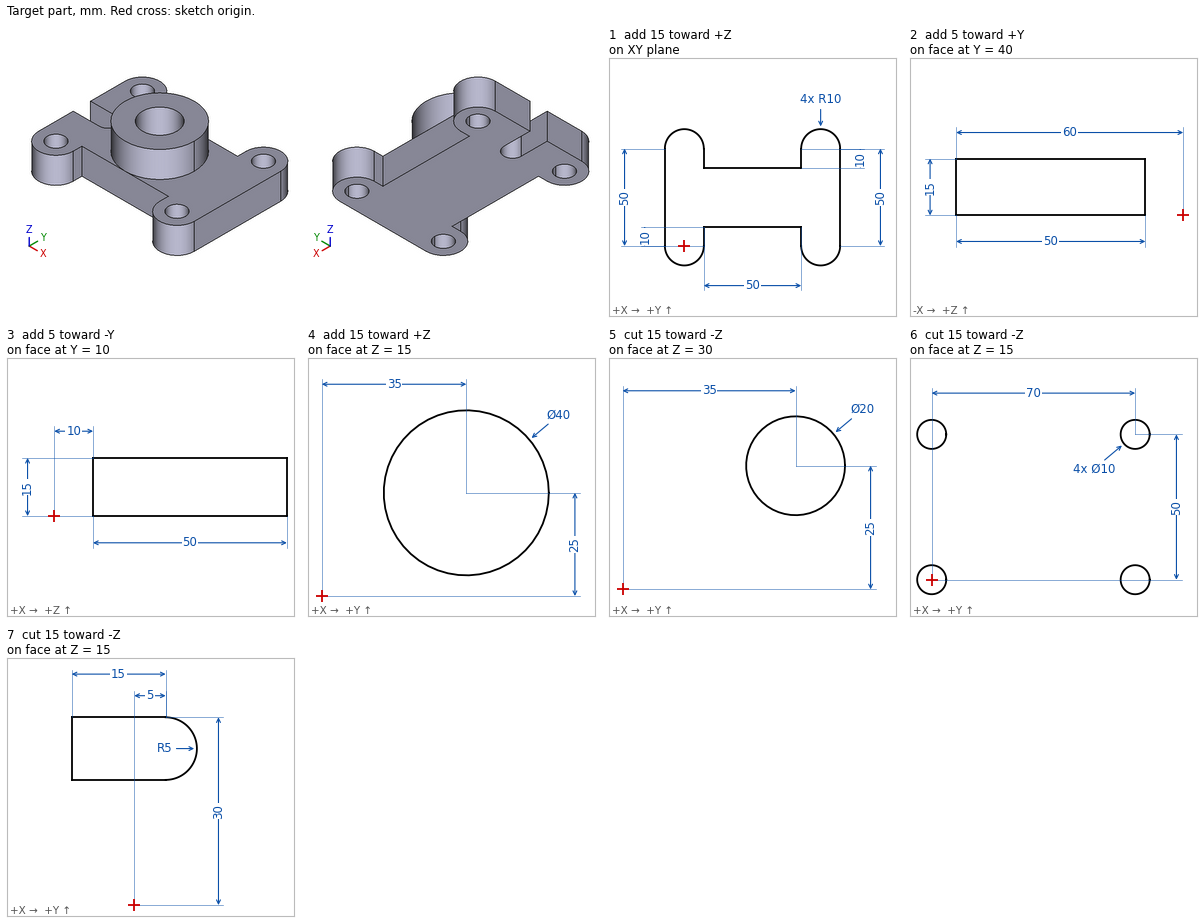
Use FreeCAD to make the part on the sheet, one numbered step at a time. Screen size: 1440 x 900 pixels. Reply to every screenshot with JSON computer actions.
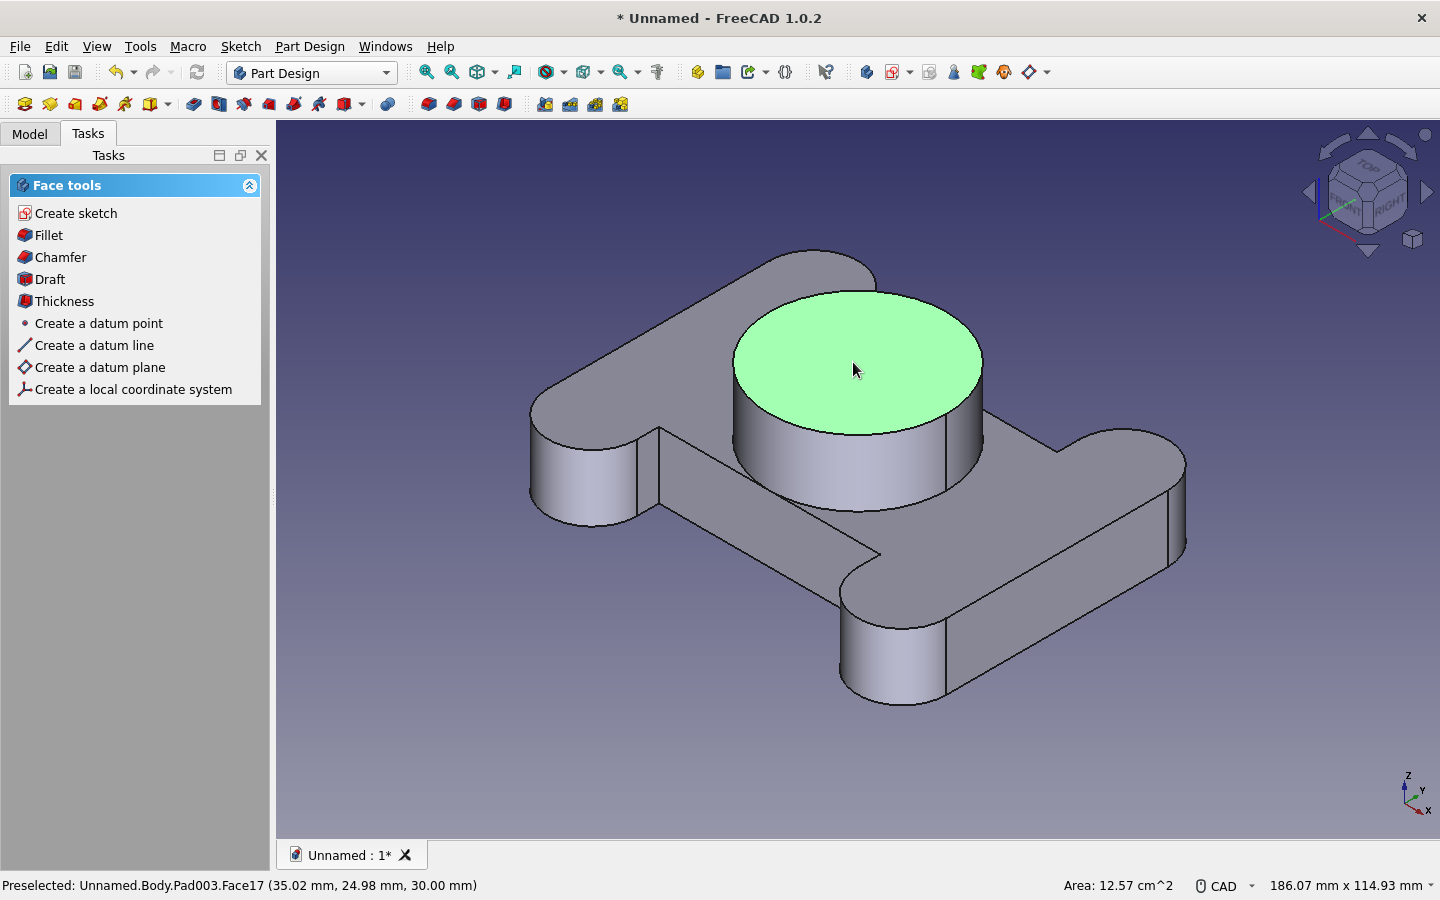
{"action": "left_click", "coordinate": [892, 72]}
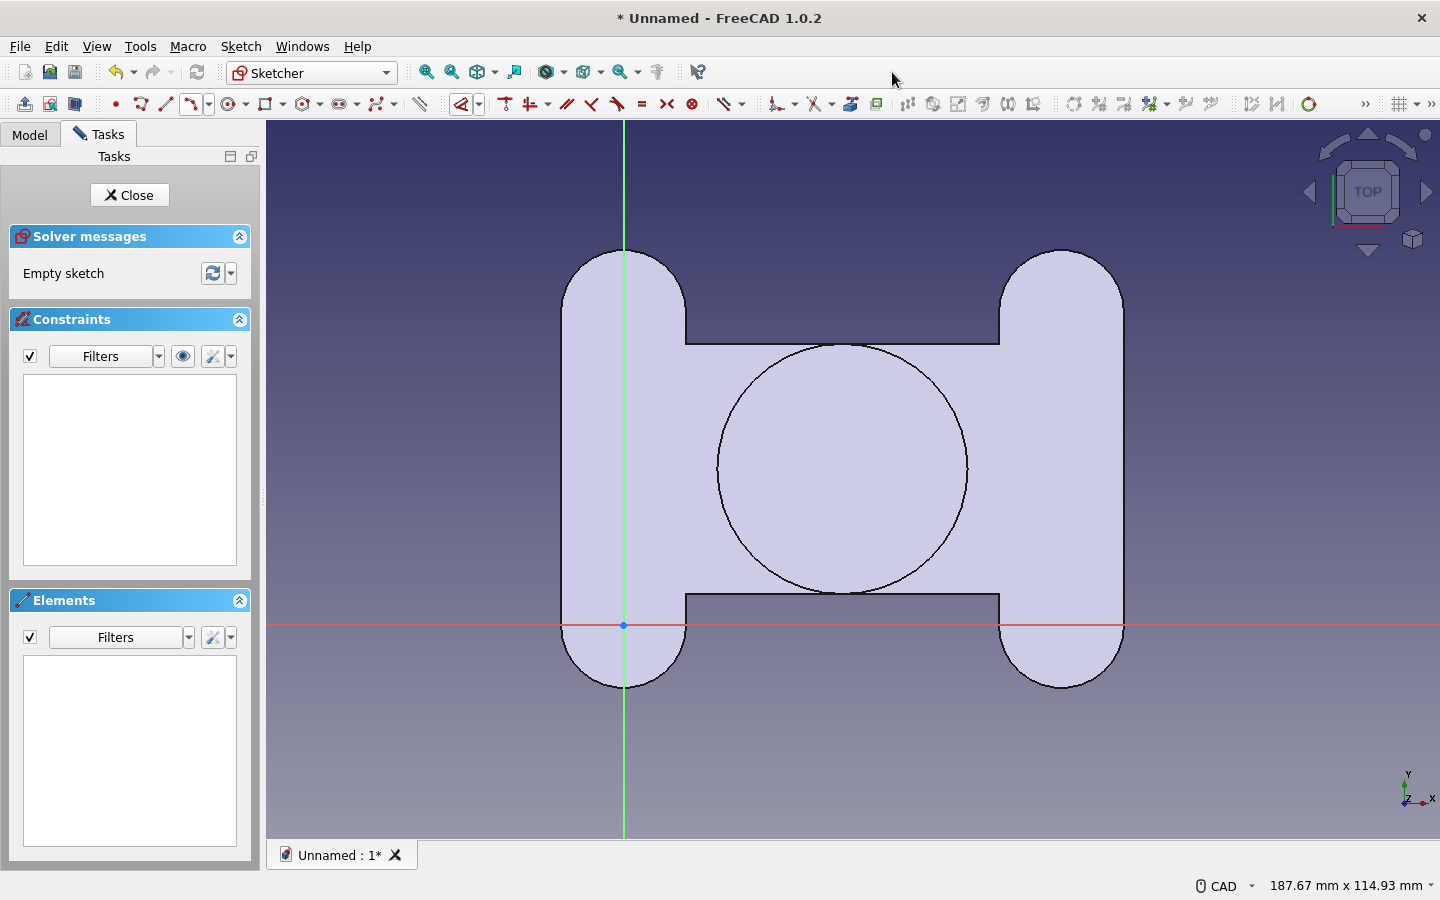
{"action": "scroll", "coordinate": [748, 546], "scroll_direction": "up", "scroll_amount": 4}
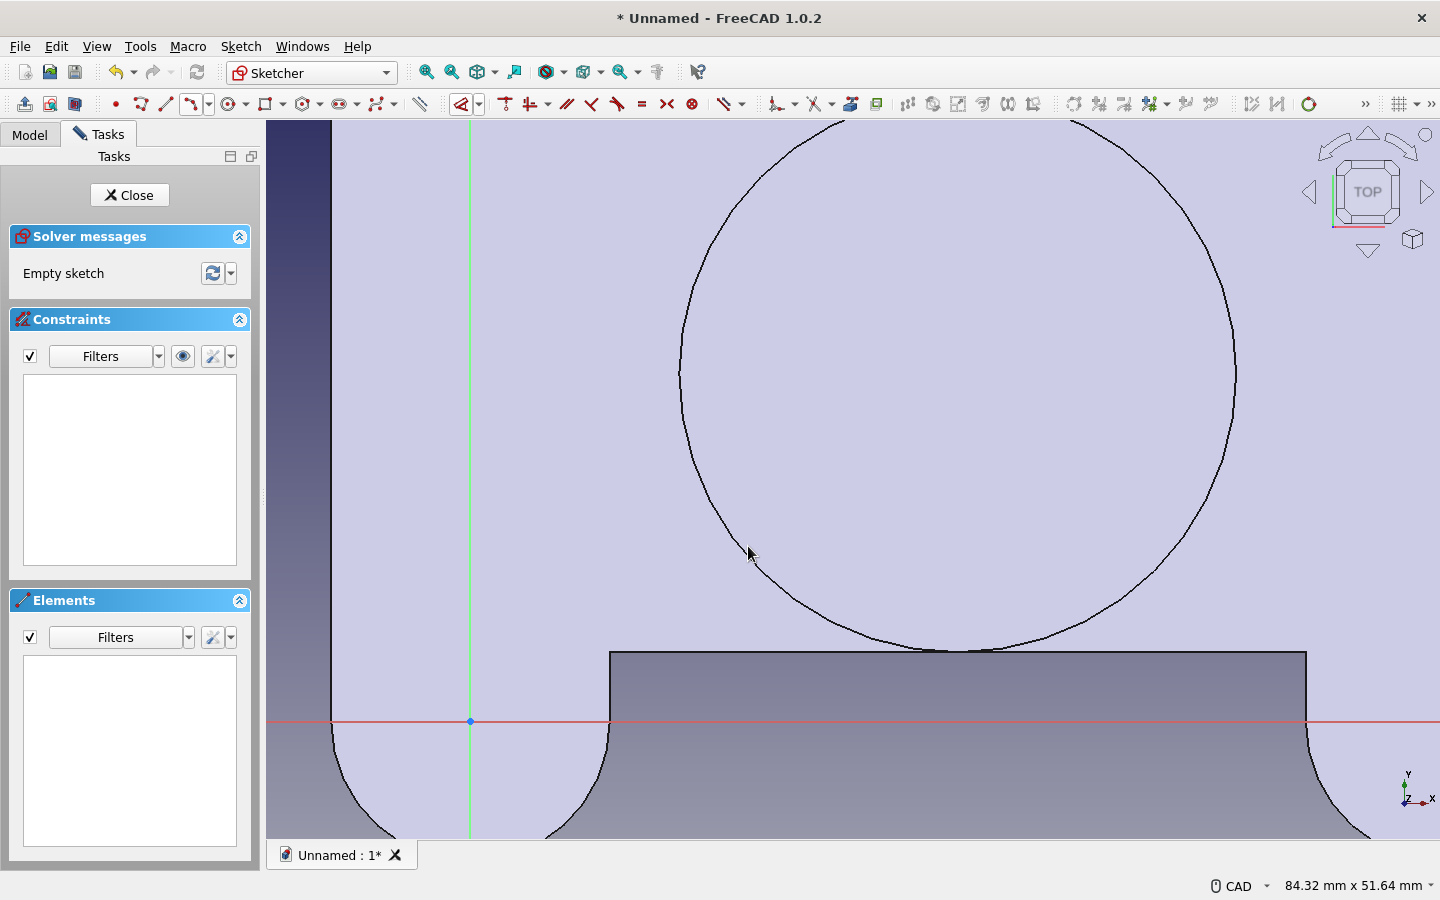
{"action": "key", "text": "g c"}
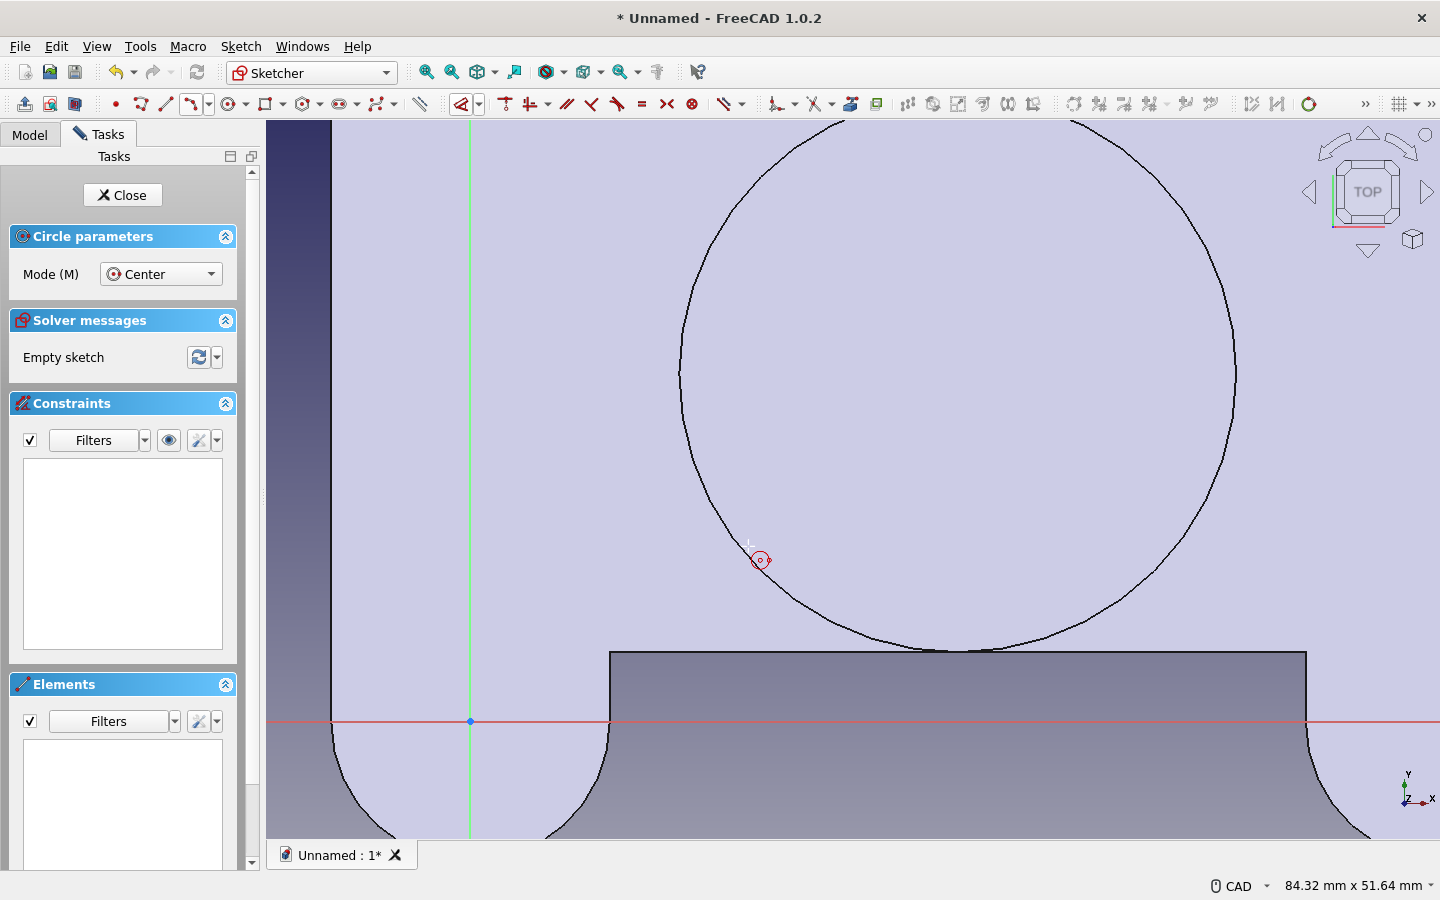
{"action": "left_click", "coordinate": [958, 374]}
{"action": "left_click", "coordinate": [1056, 275]}
{"action": "key", "text": "Escape"}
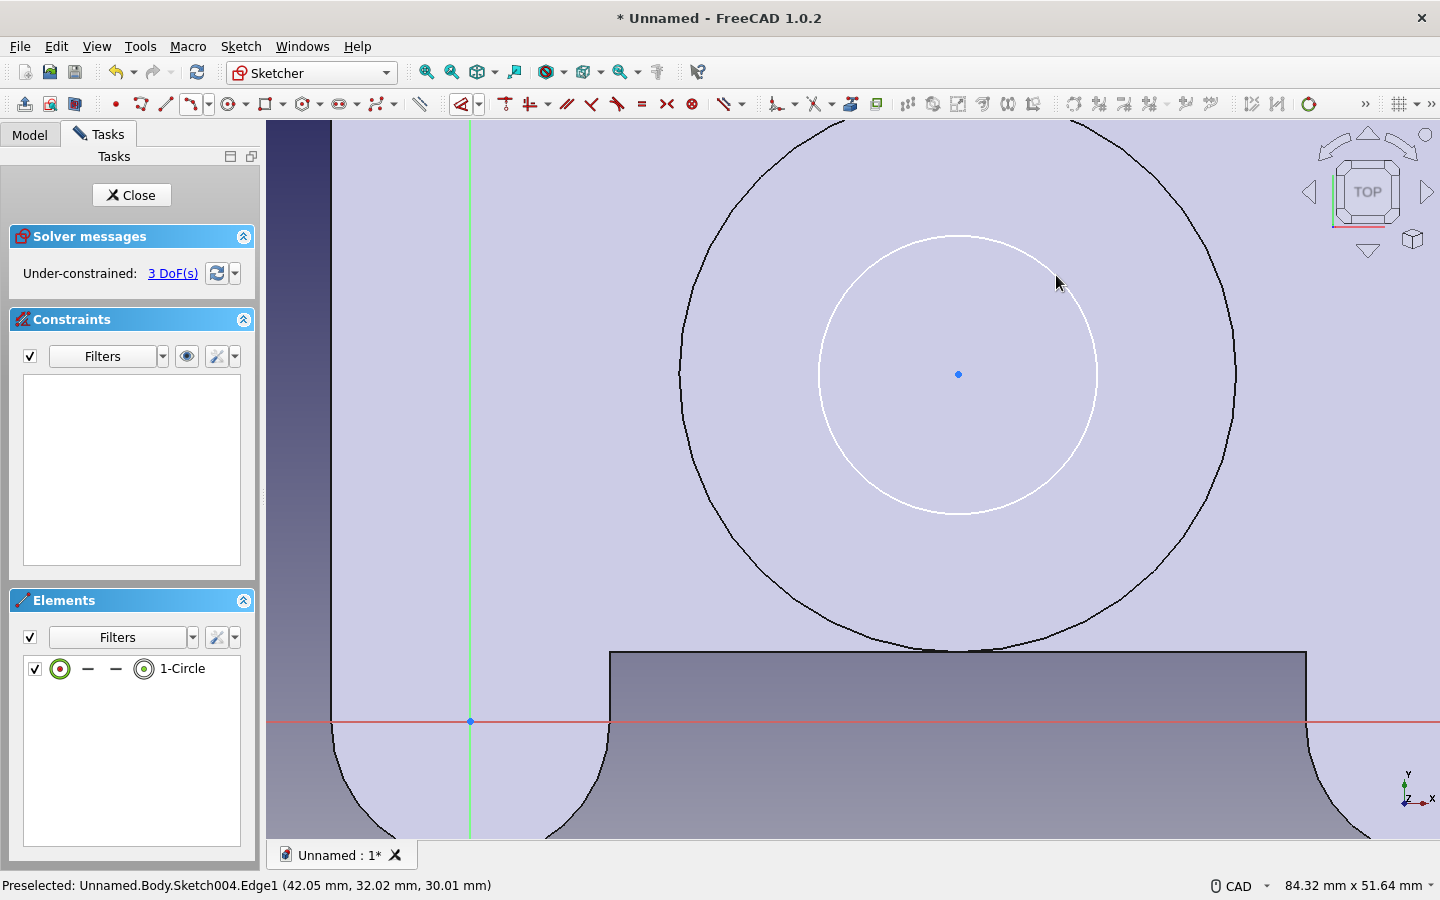
{"action": "left_click", "coordinate": [1056, 276]}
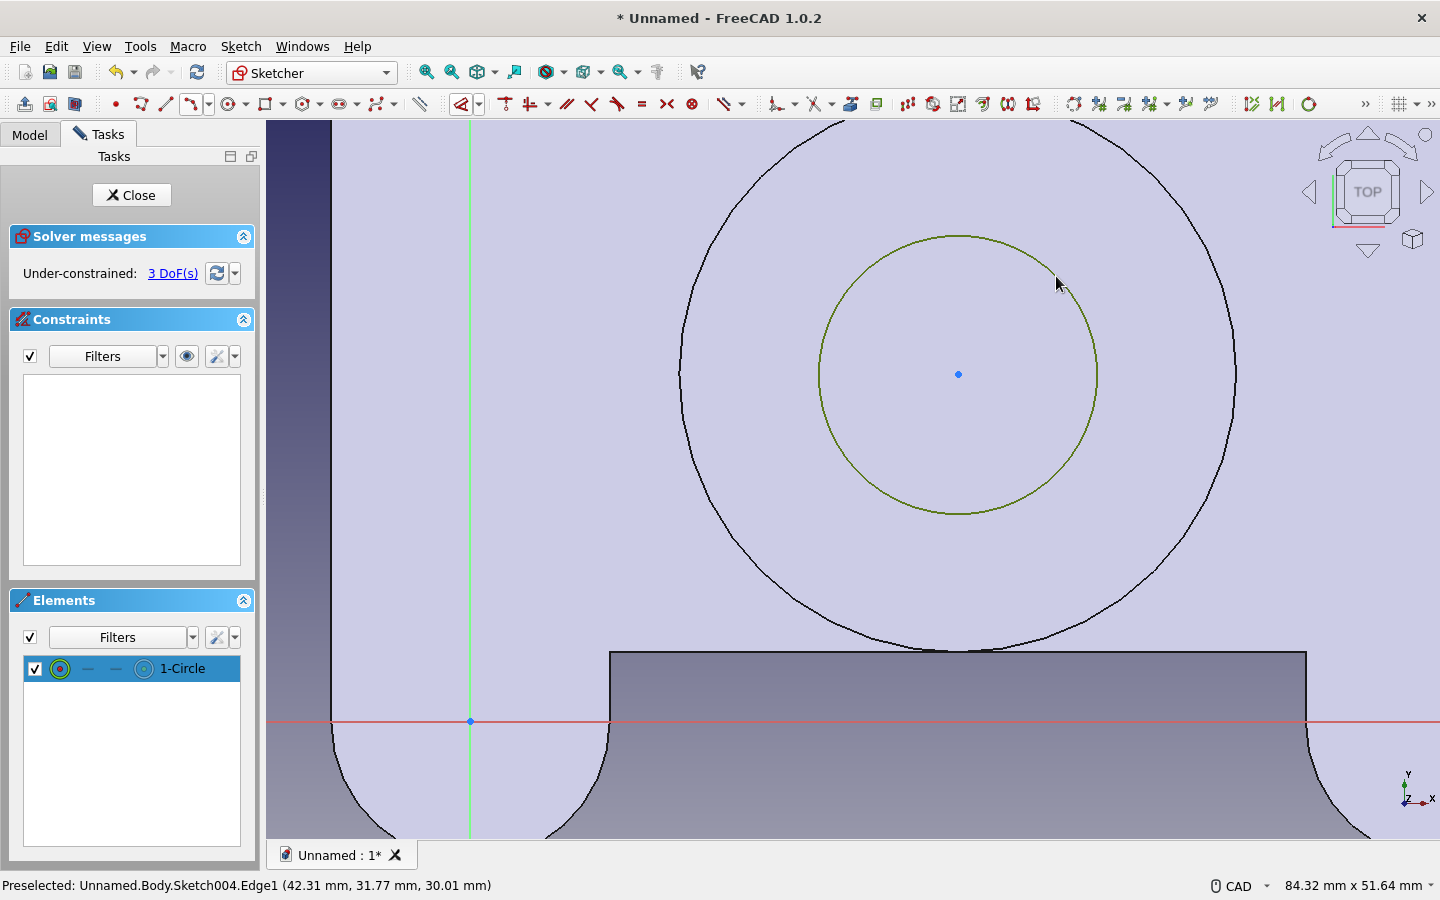
{"action": "key", "text": "k o"}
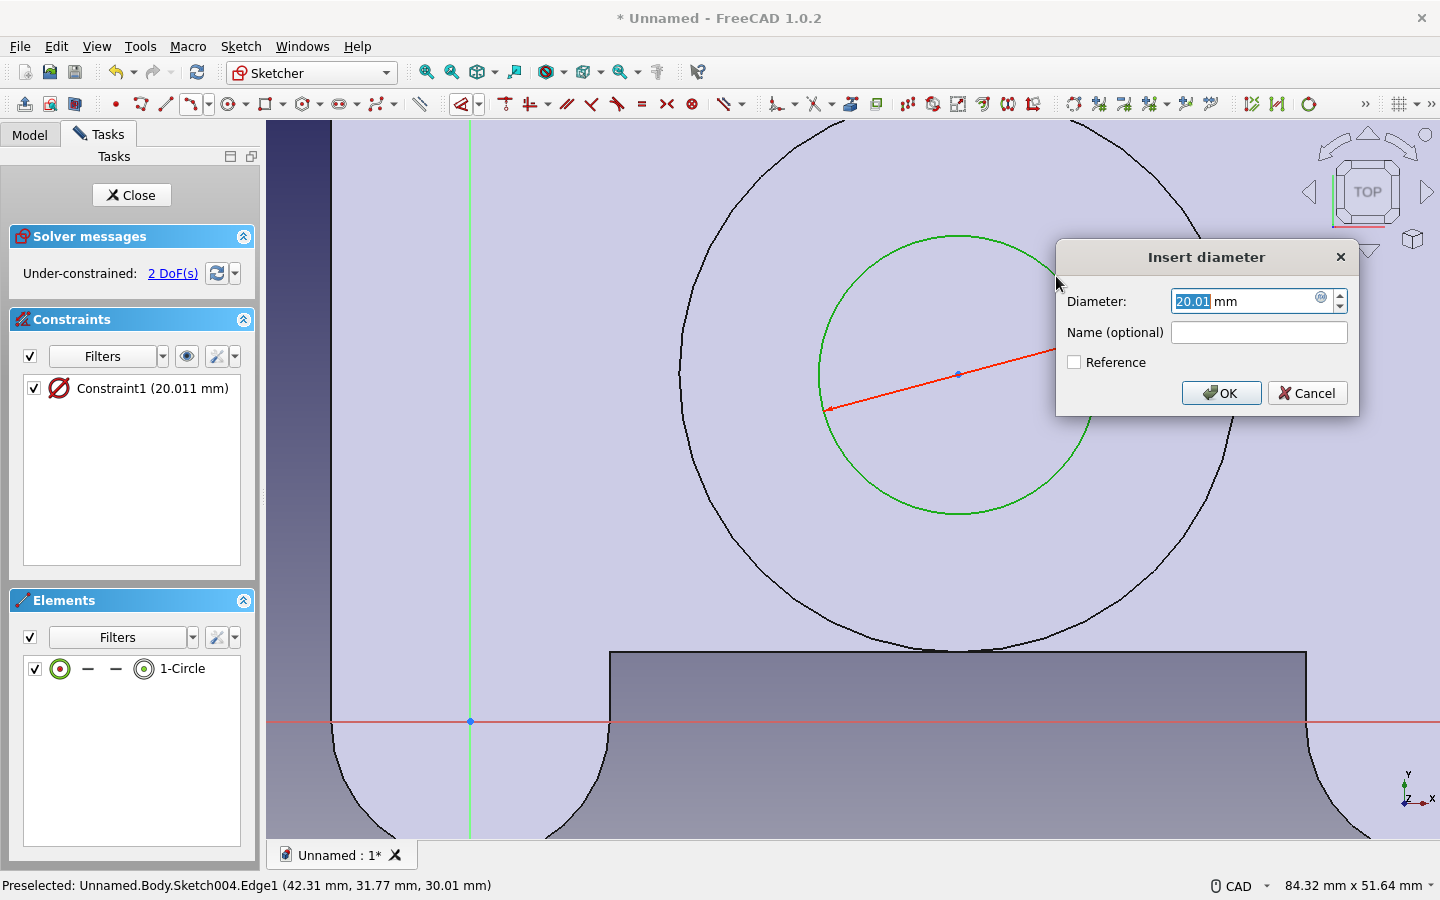
{"action": "type", "text": "20"}
{"action": "key", "text": "Return"}